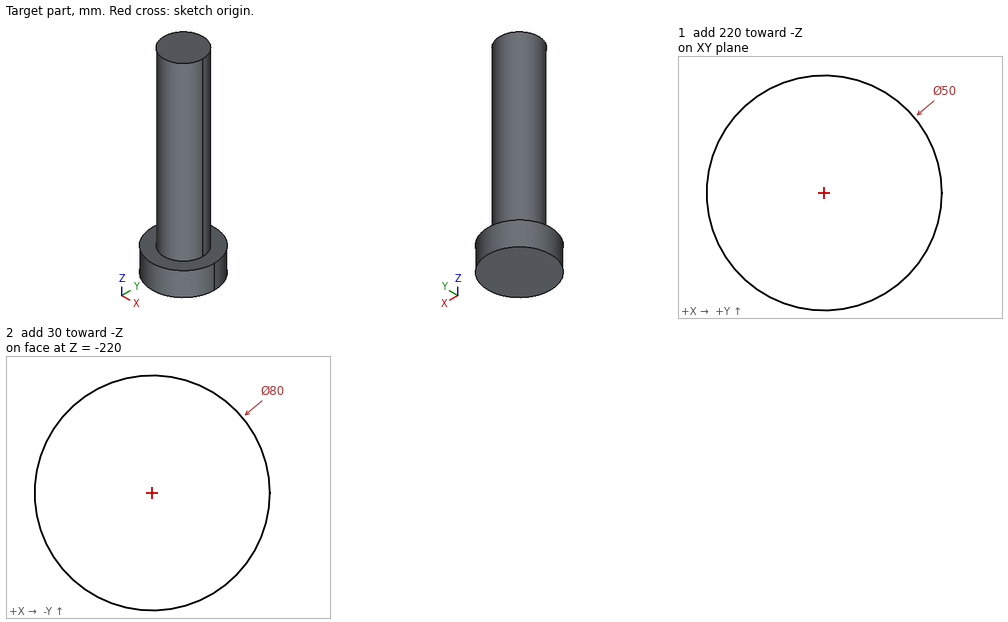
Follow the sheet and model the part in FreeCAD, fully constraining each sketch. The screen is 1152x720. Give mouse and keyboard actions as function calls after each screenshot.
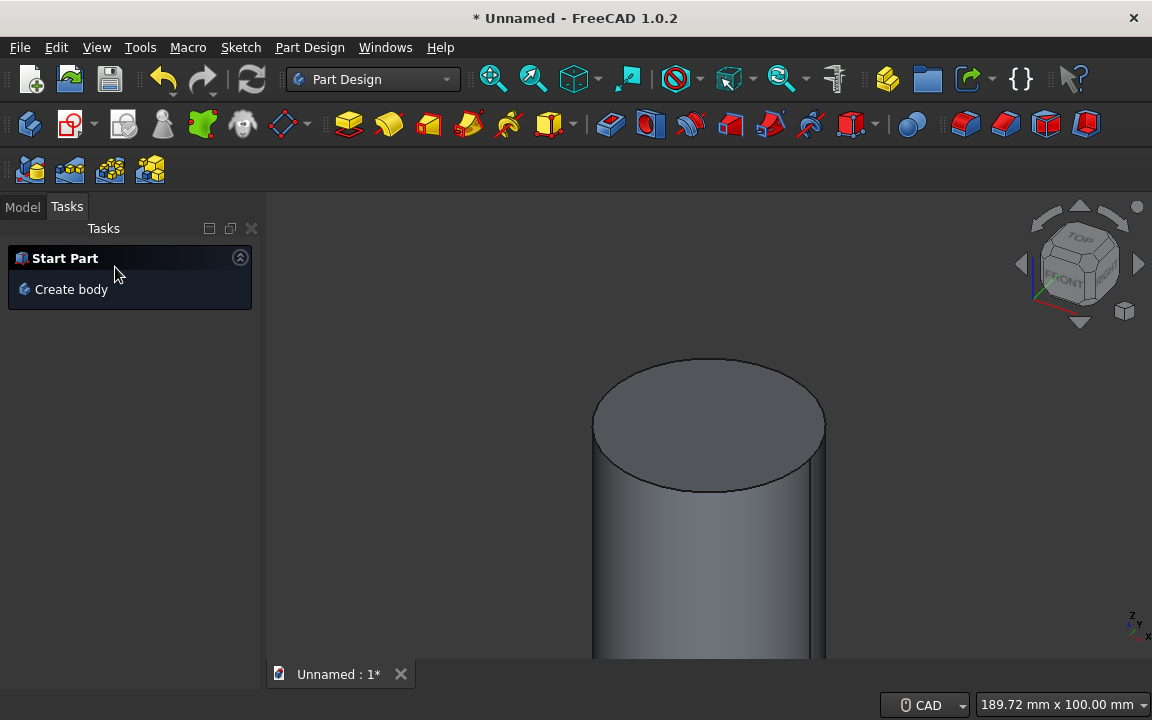
click(494, 80)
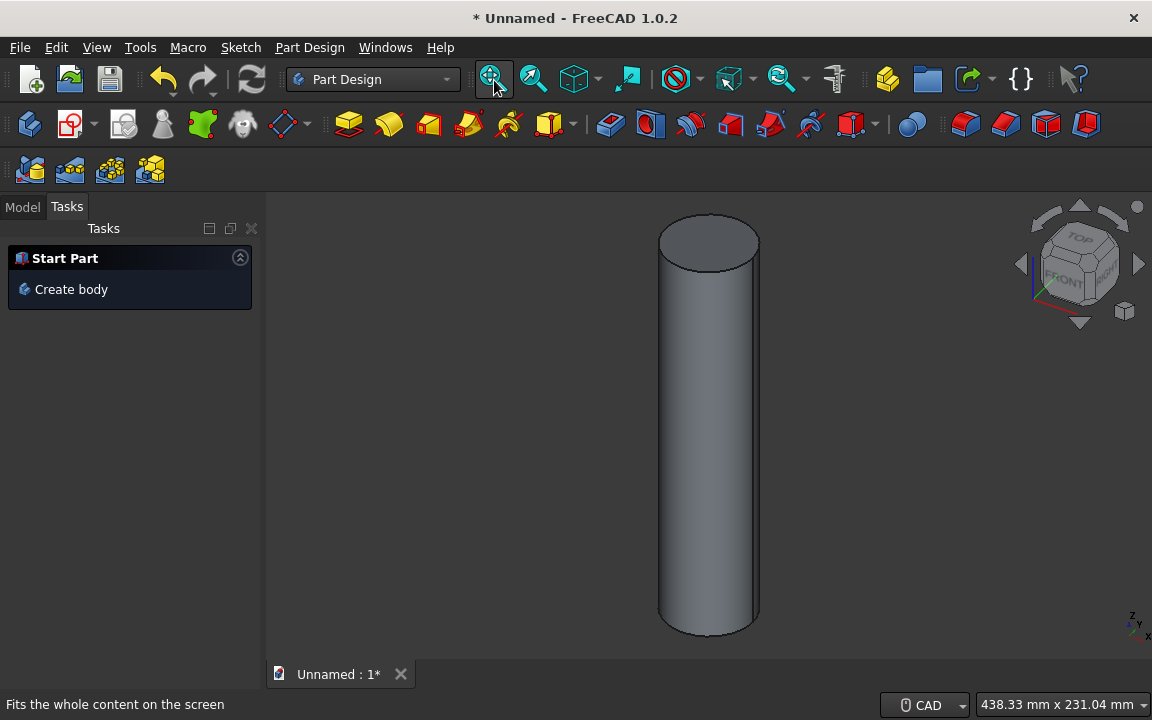
key(5)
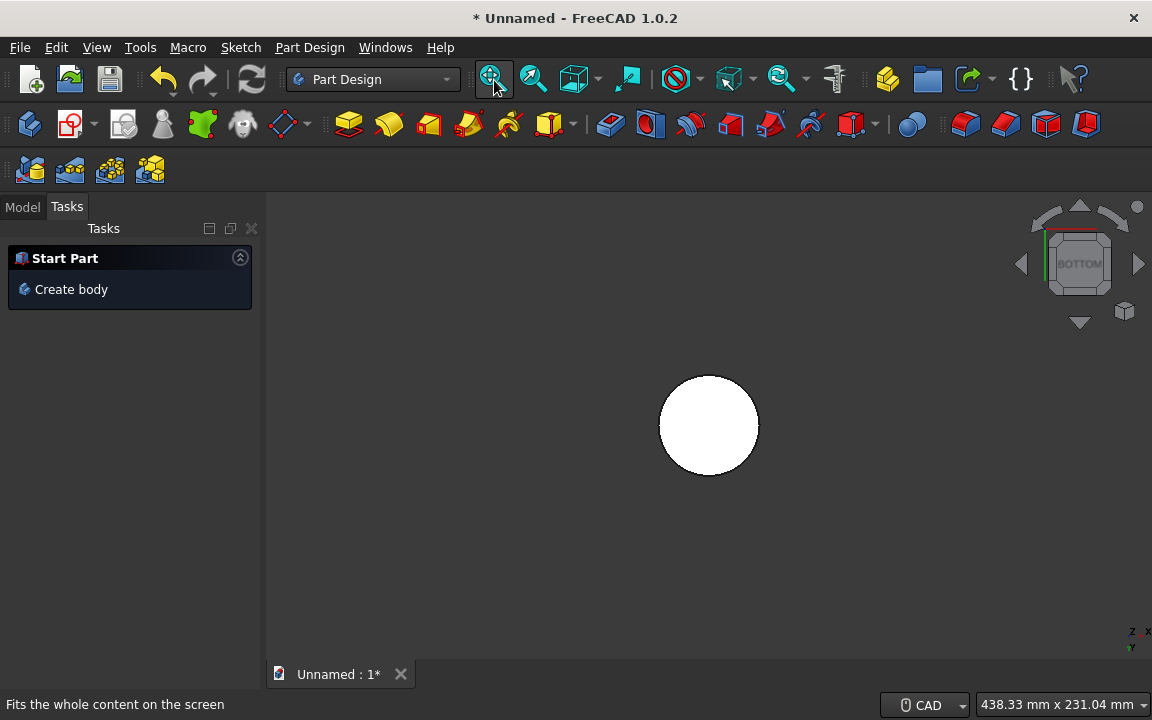
click(494, 80)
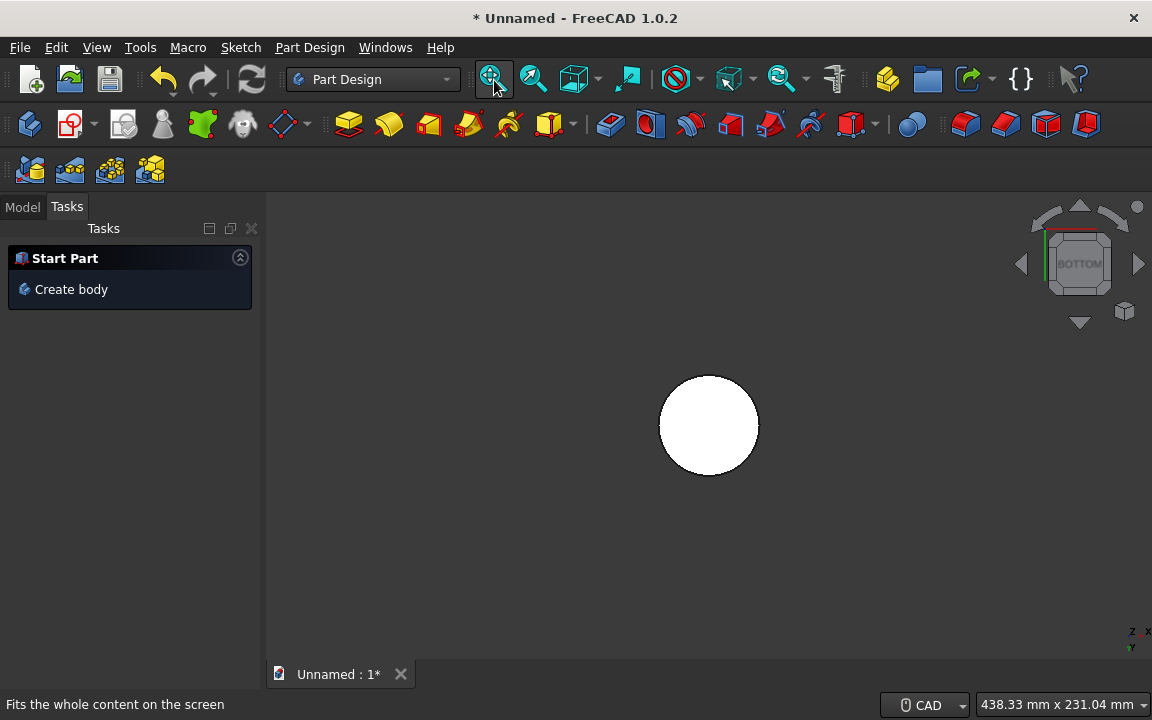
click(709, 424)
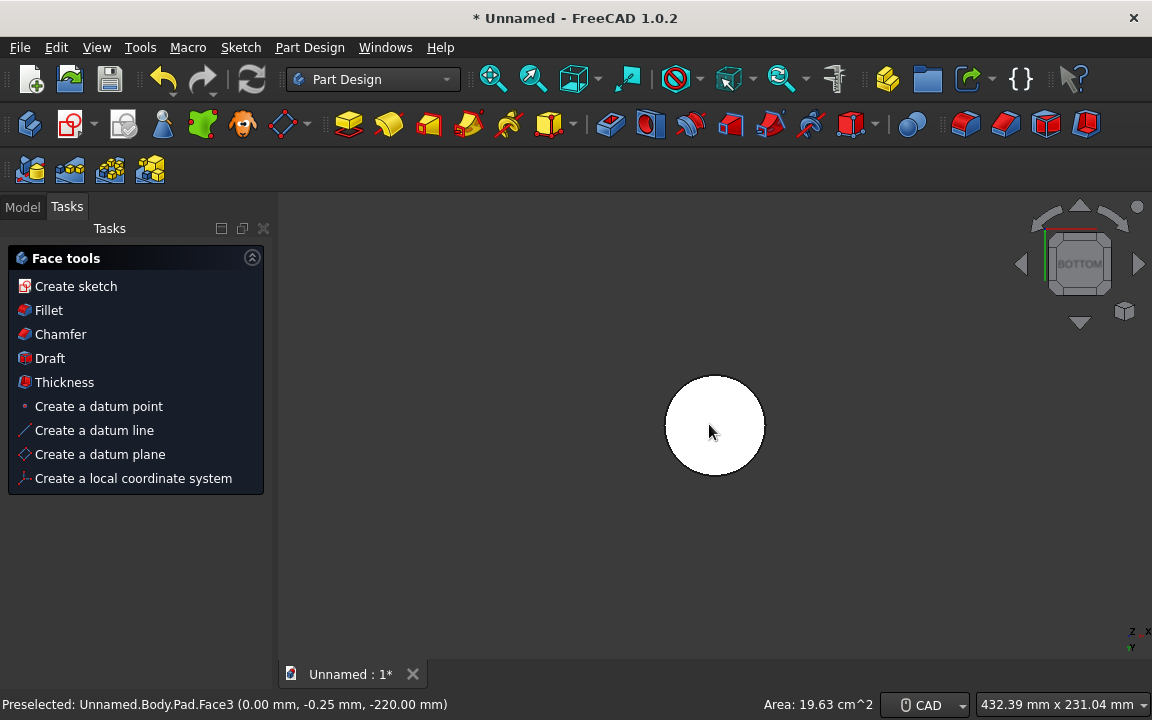
click(70, 124)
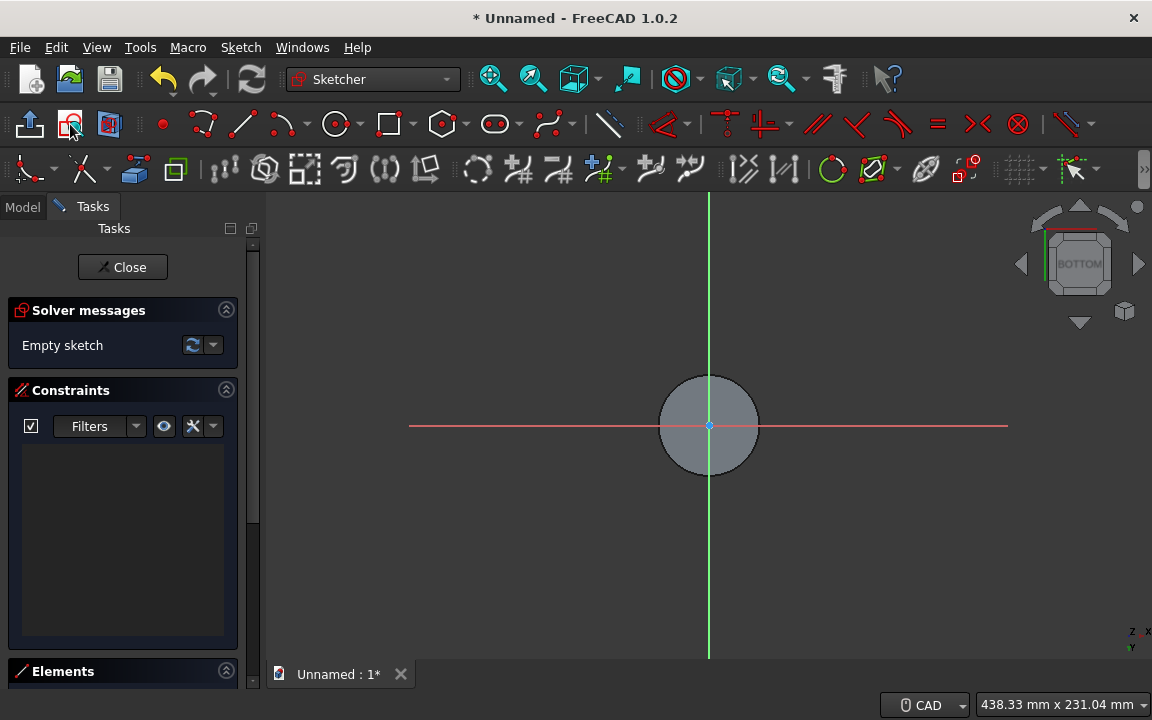
scroll(792, 426, up, 3)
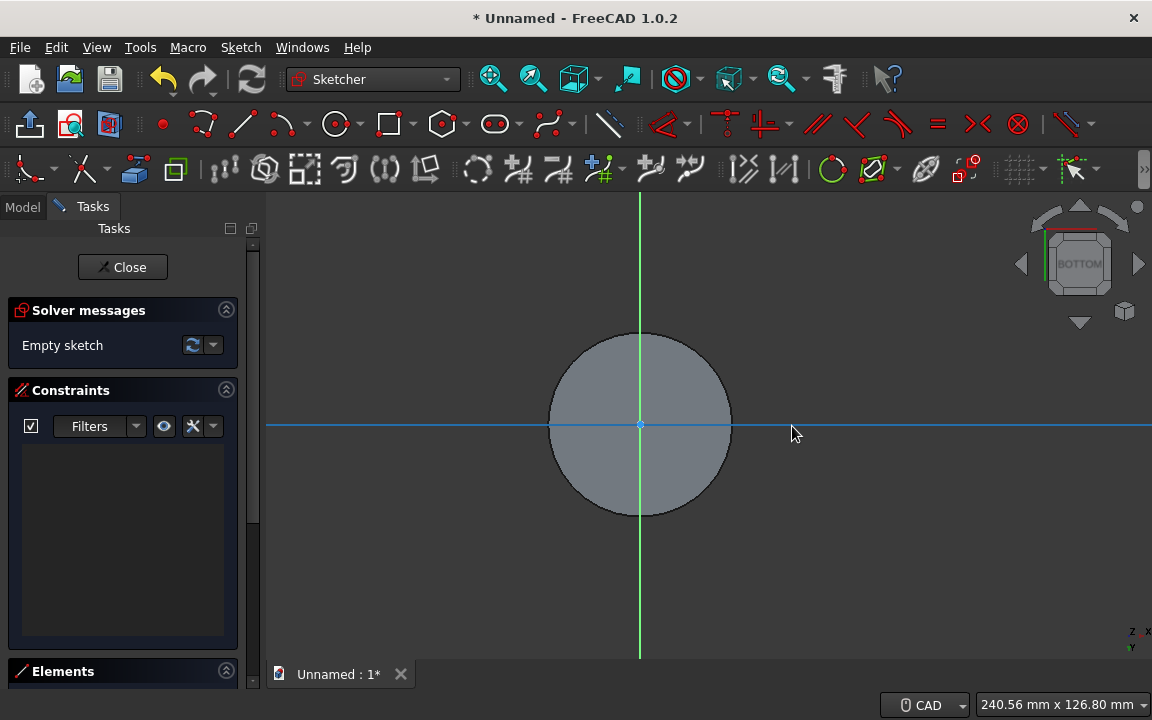
click(336, 124)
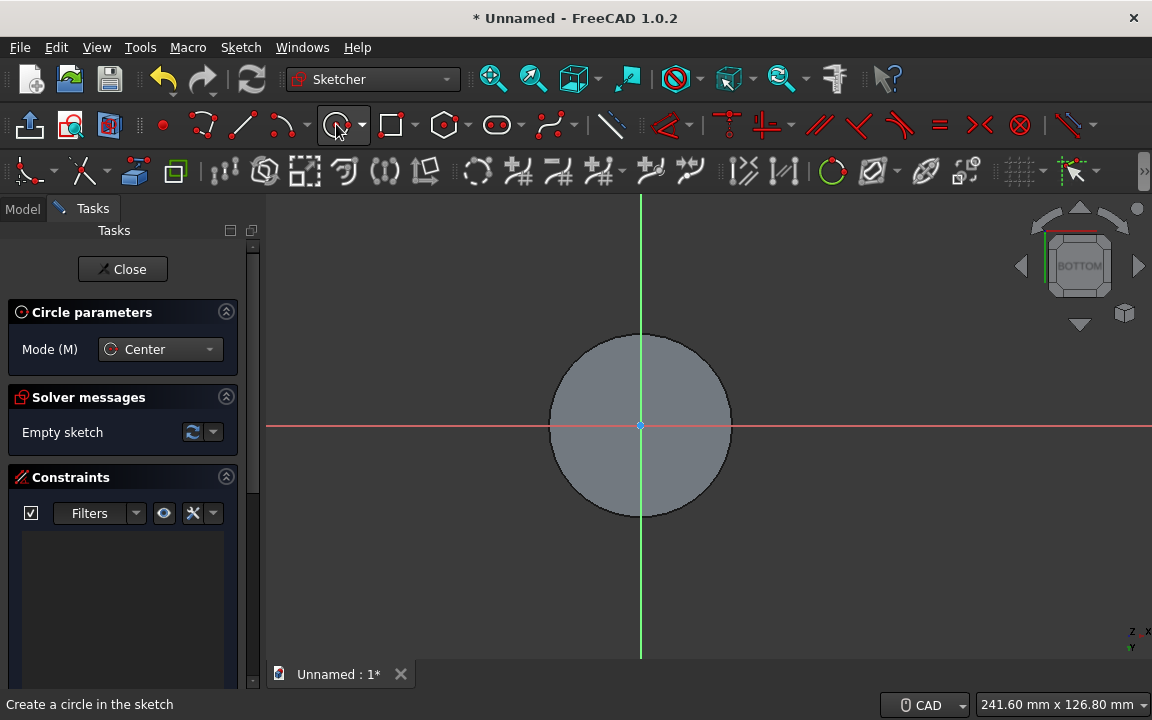
click(641, 426)
move(744, 322)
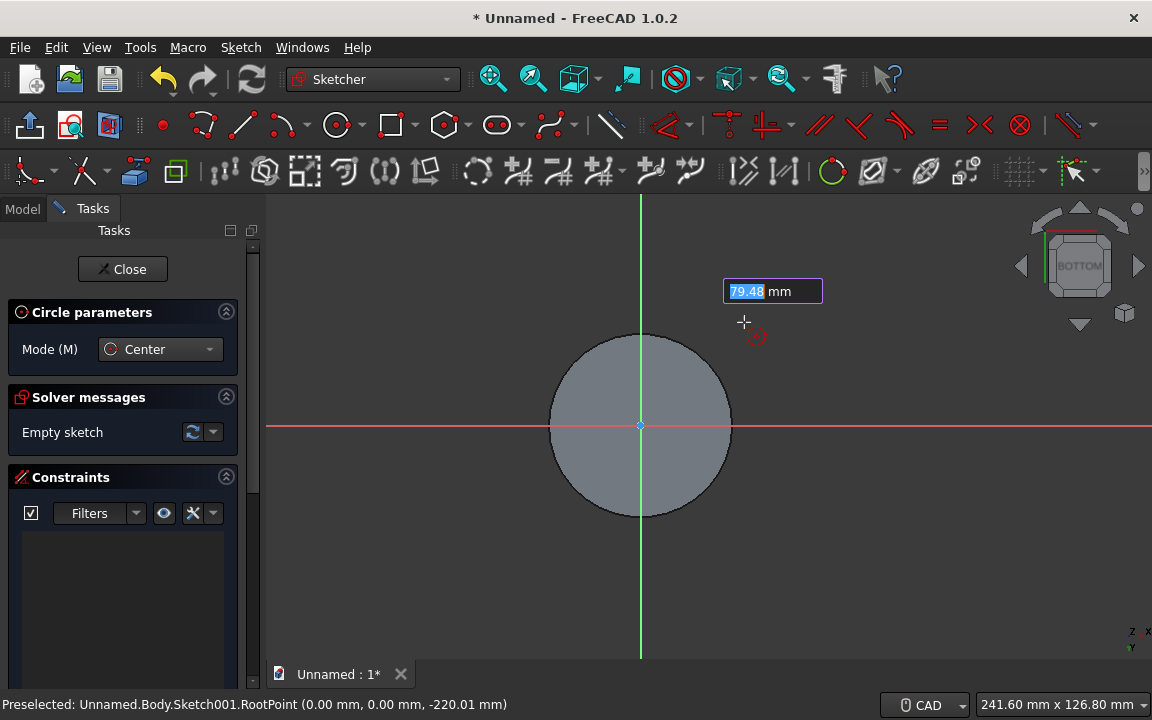
text(80)
key(Return)
key(Escape)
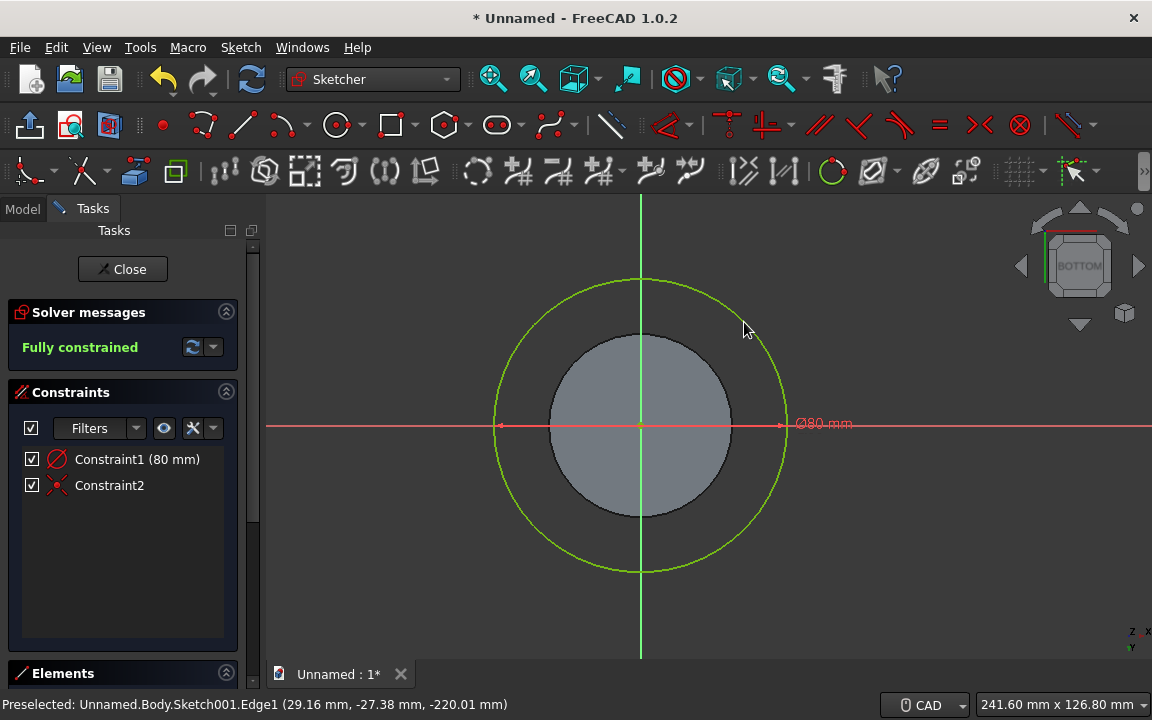
click(123, 269)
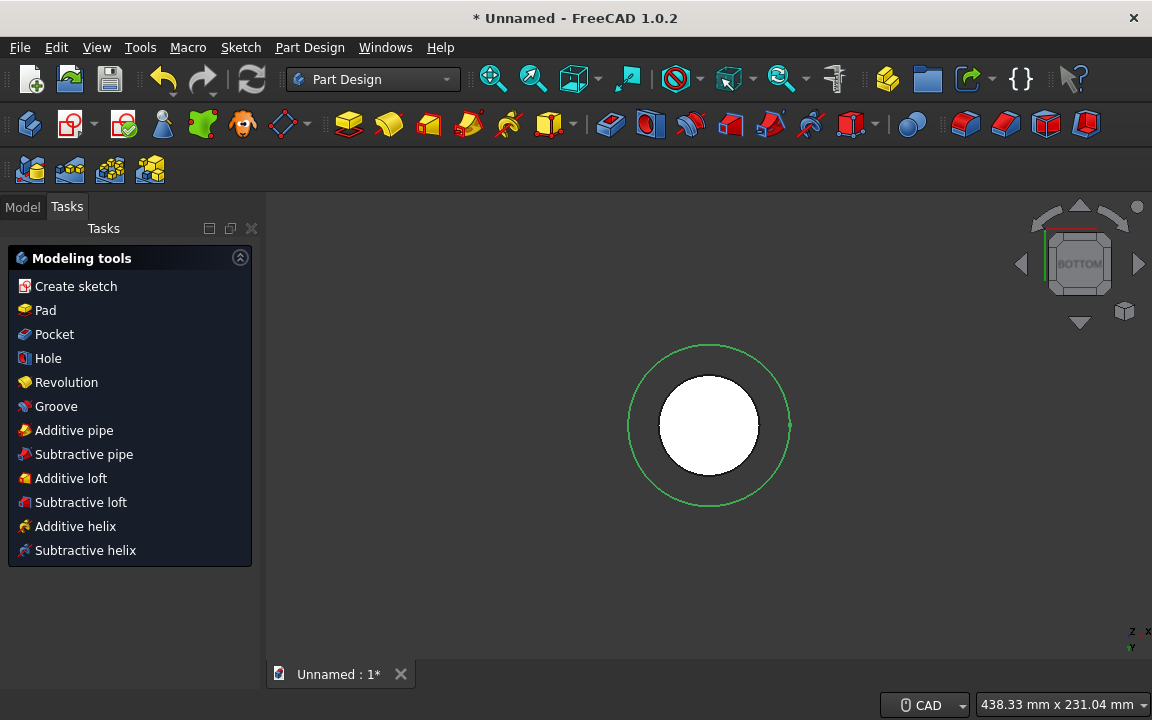
click(350, 124)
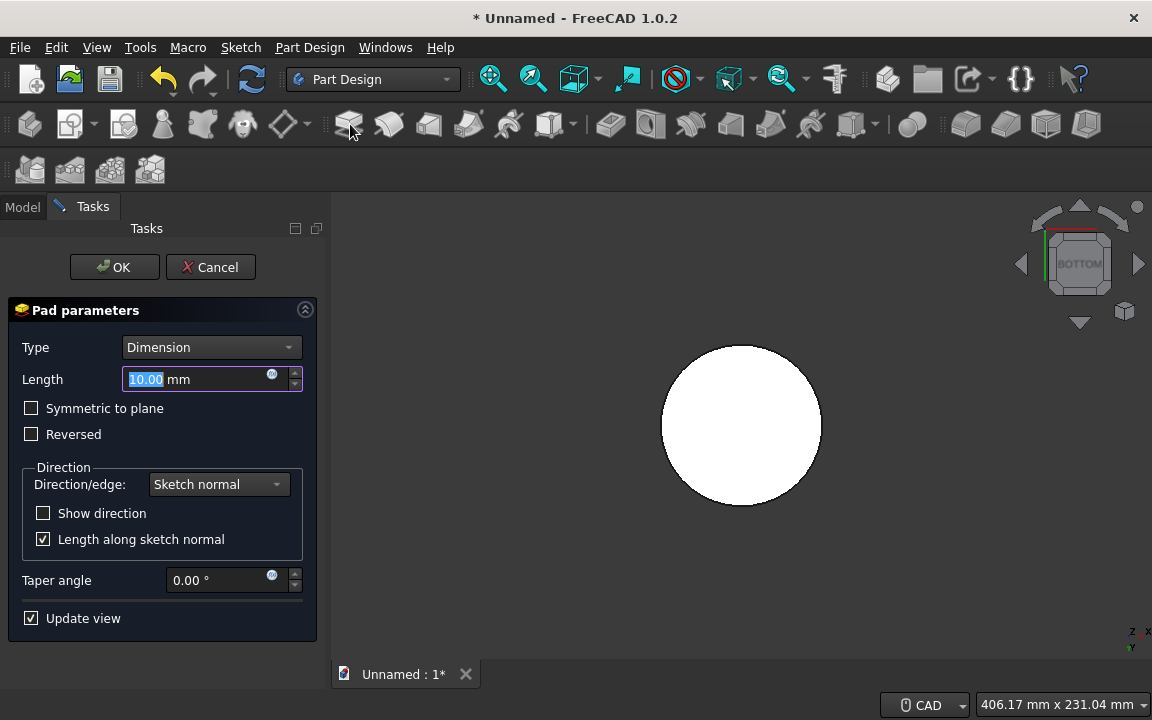
text(30)
key(Tab)